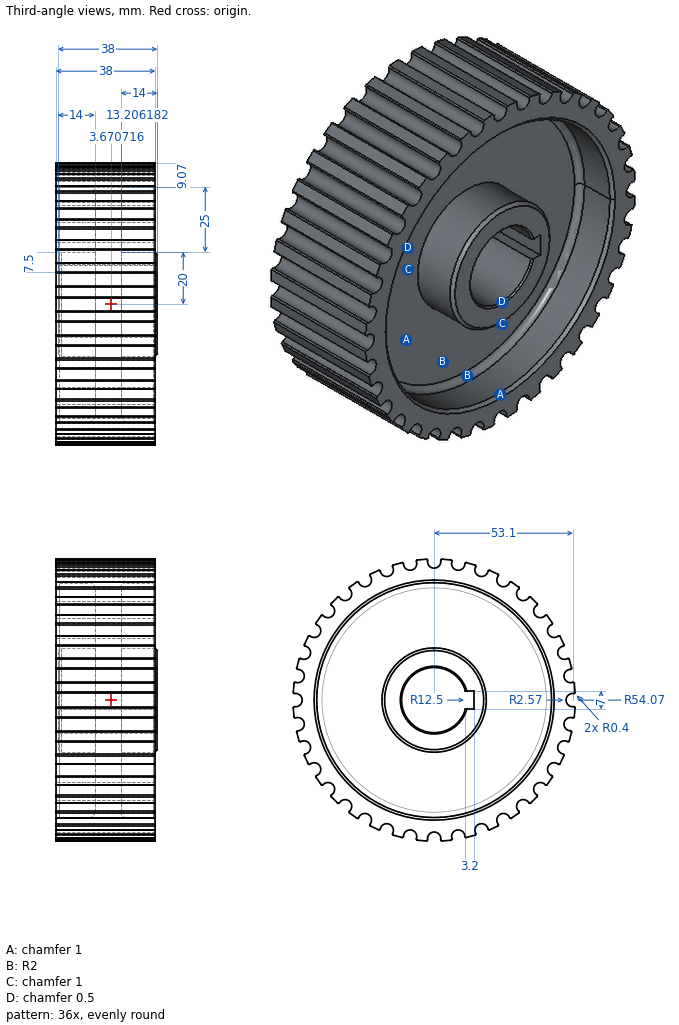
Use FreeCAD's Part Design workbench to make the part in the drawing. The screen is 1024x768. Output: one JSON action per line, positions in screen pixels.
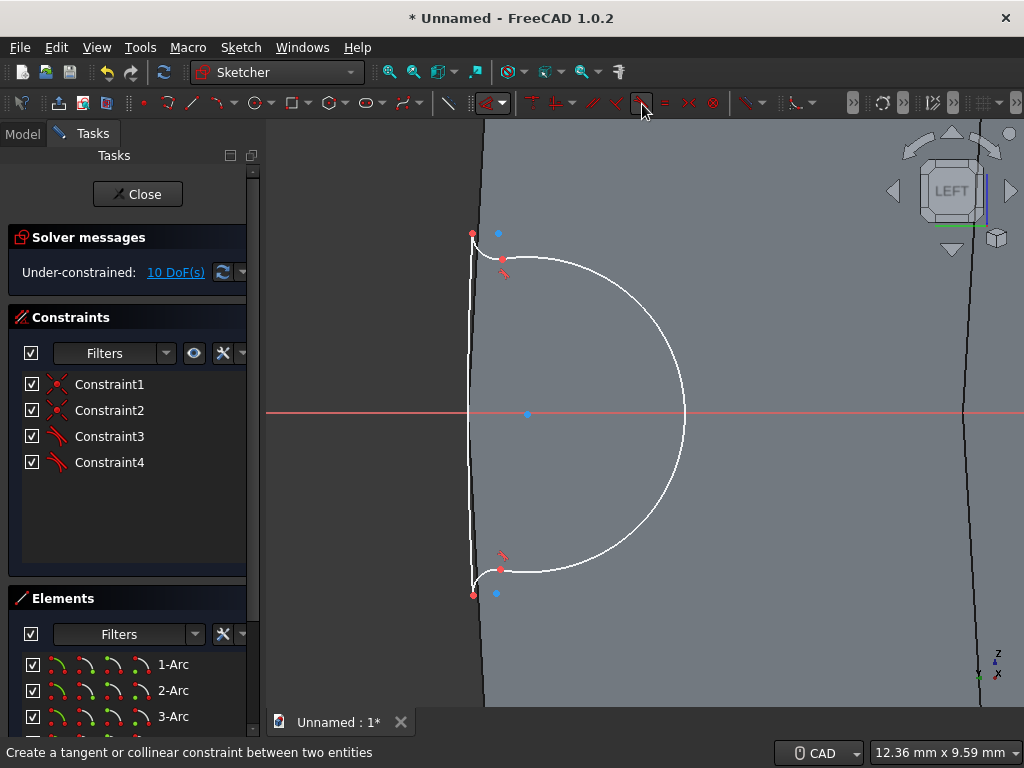
{"action": "left_click", "coordinate": [489, 258]}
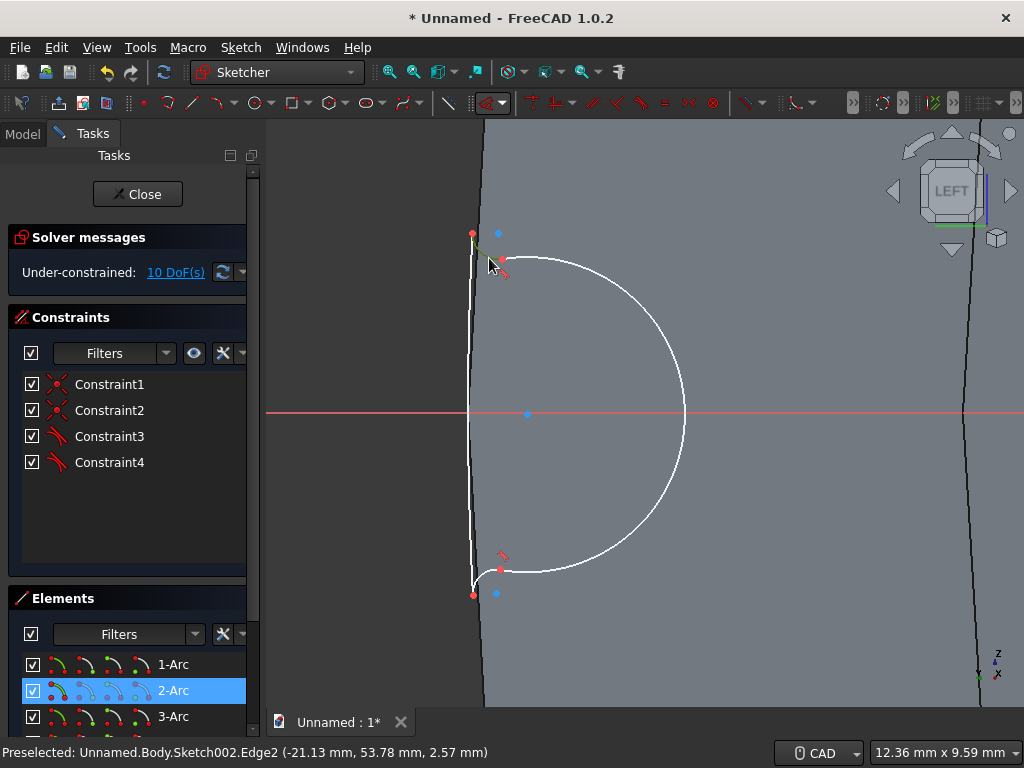
{"action": "left_click", "coordinate": [469, 342]}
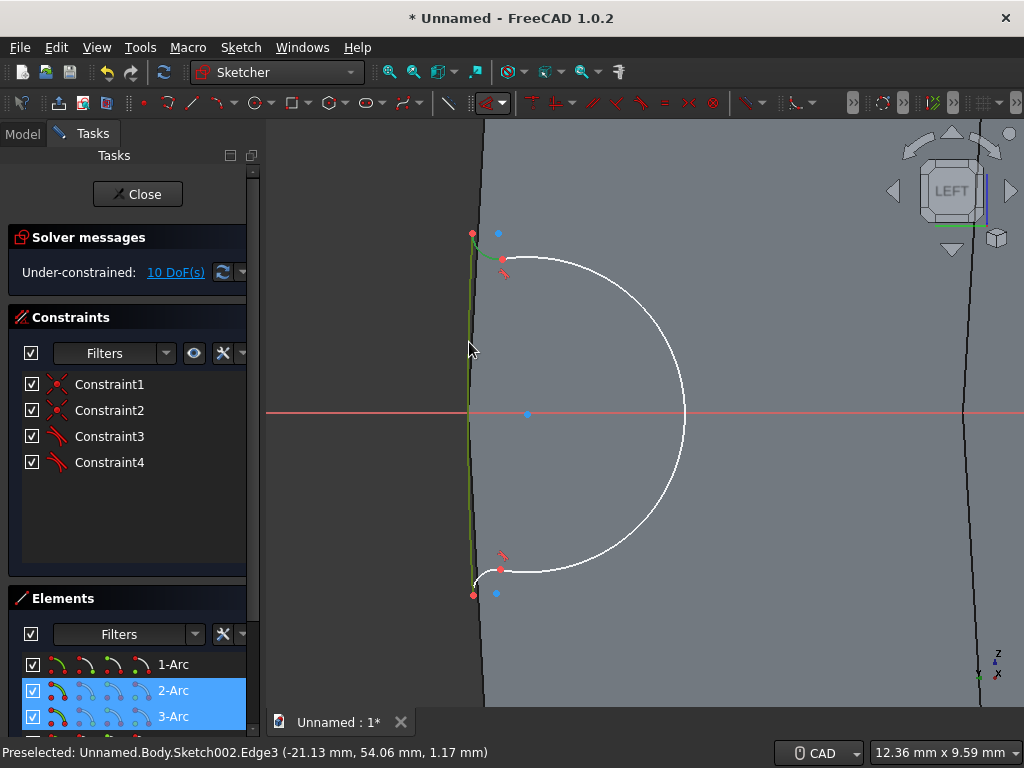
{"action": "key", "text": "t"}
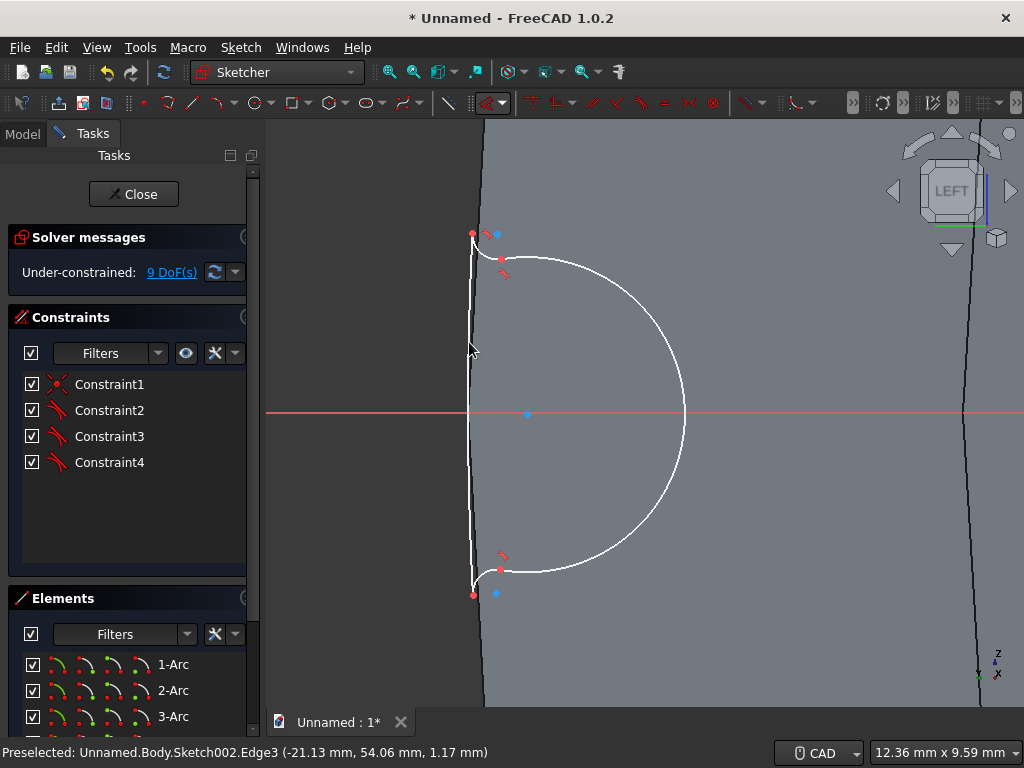
{"action": "left_click", "coordinate": [469, 342]}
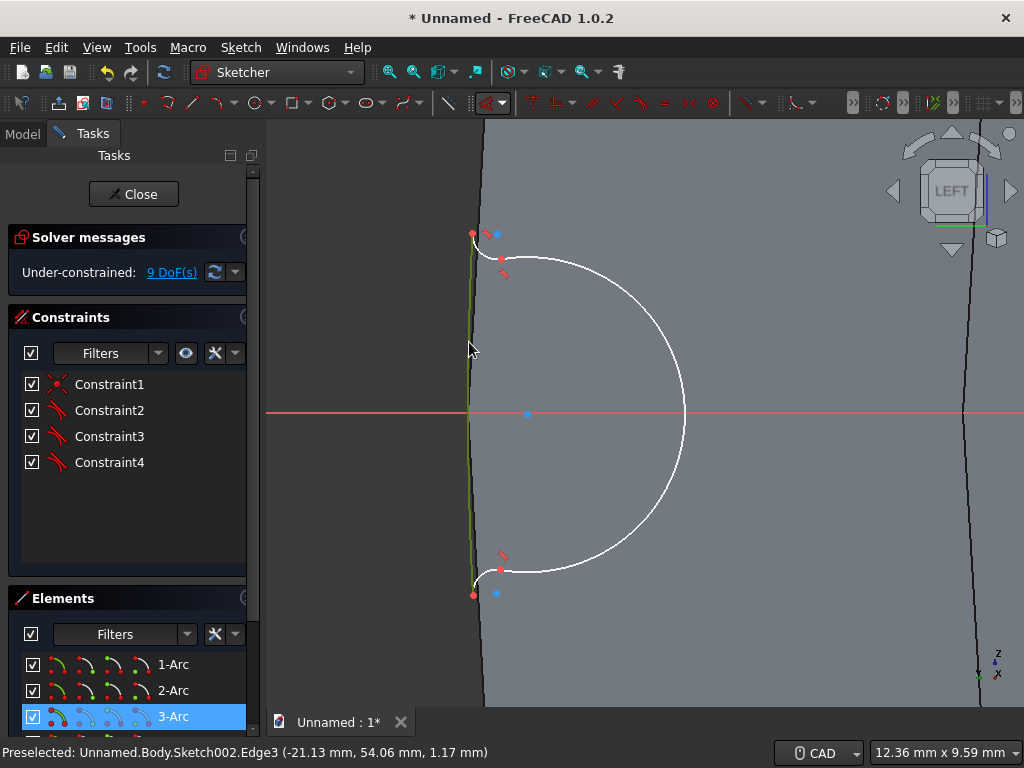
{"action": "left_click", "coordinate": [488, 571]}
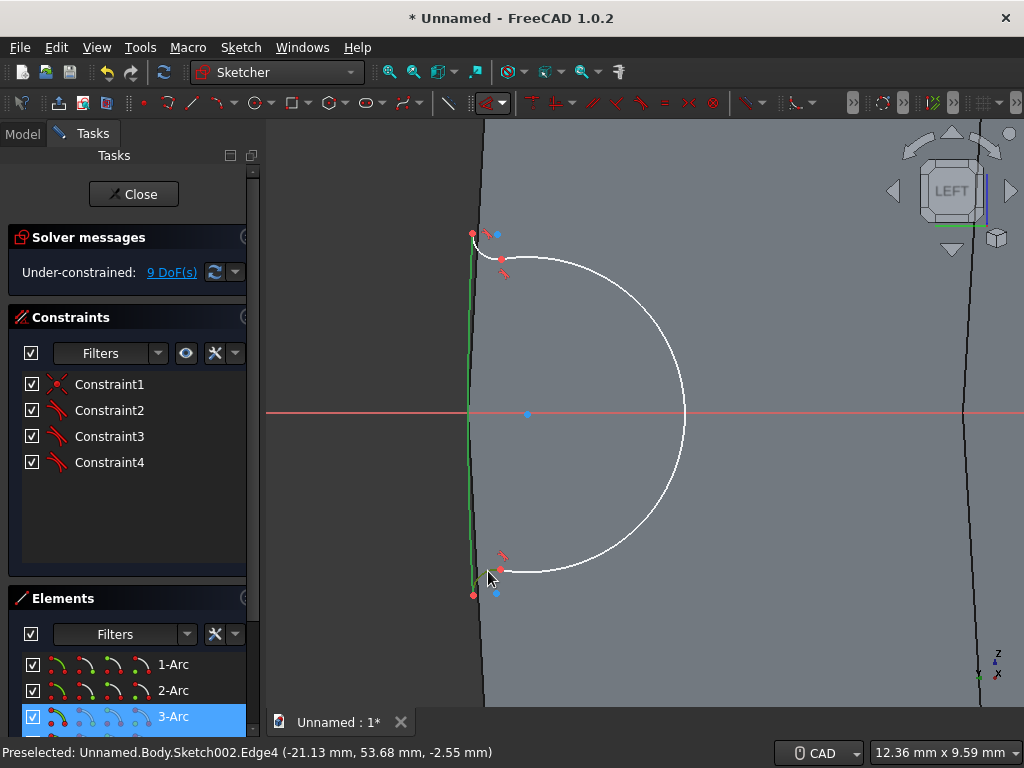
{"action": "key", "text": "t"}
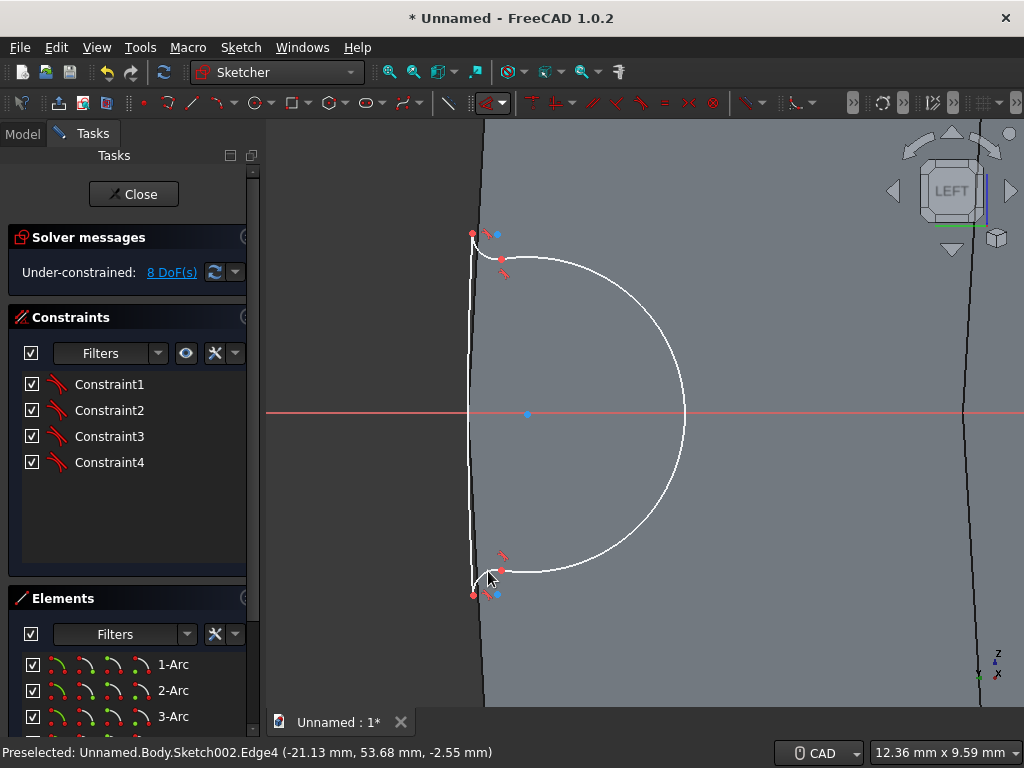
{"action": "scroll", "coordinate": [378, 413], "scroll_direction": "down", "scroll_amount": 11}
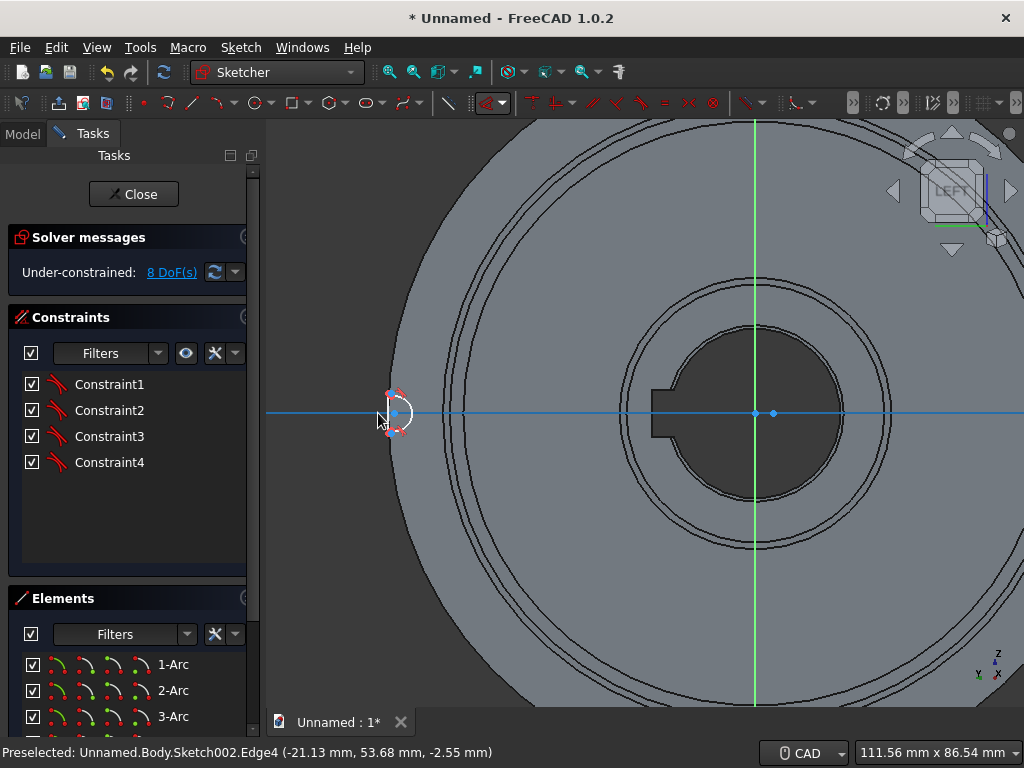
{"action": "scroll", "coordinate": [764, 413], "scroll_direction": "up", "scroll_amount": 14}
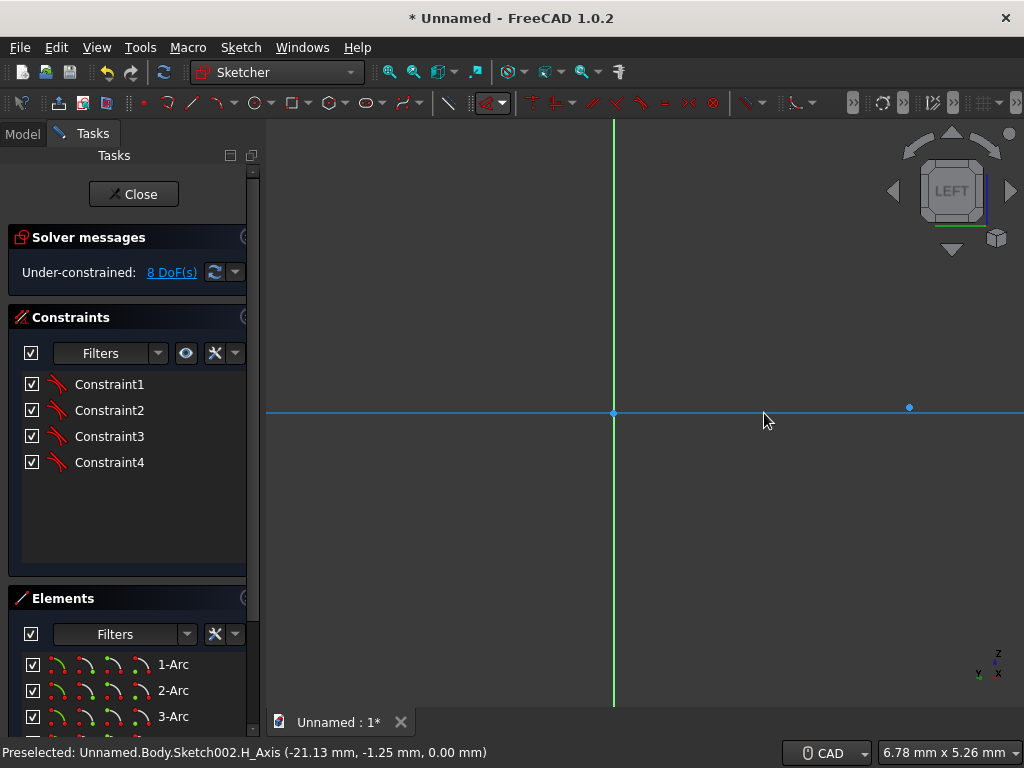
{"action": "left_click_drag", "start_coordinate": [604, 397], "coordinate": [919, 423]}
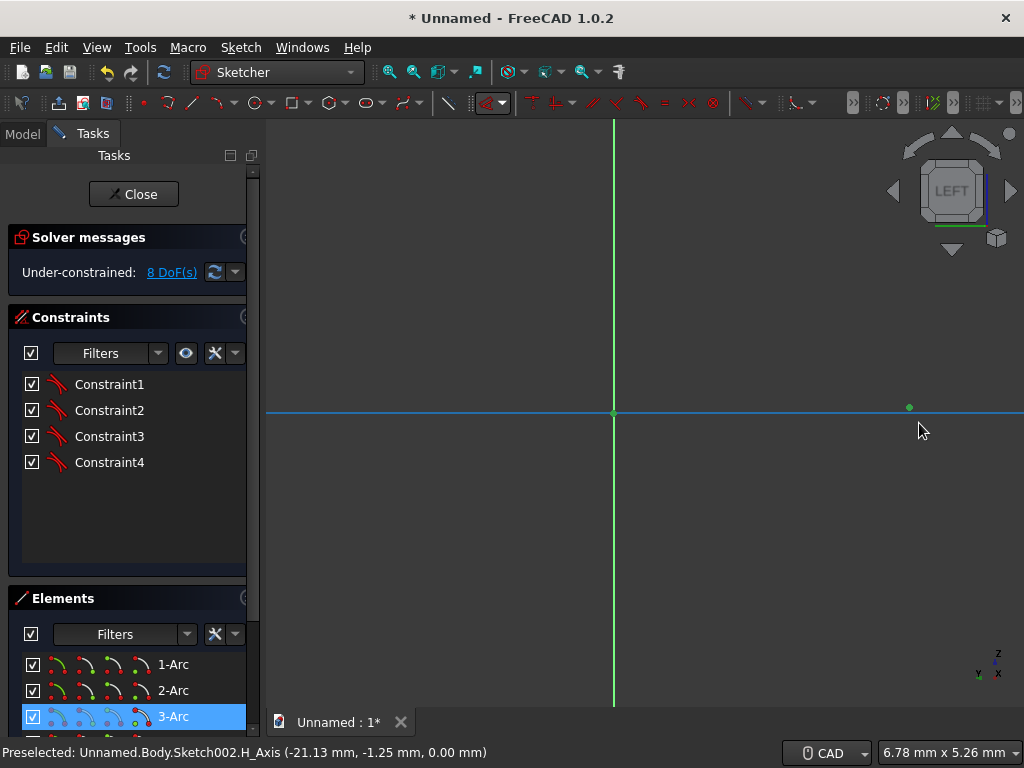
{"action": "left_click", "coordinate": [532, 104]}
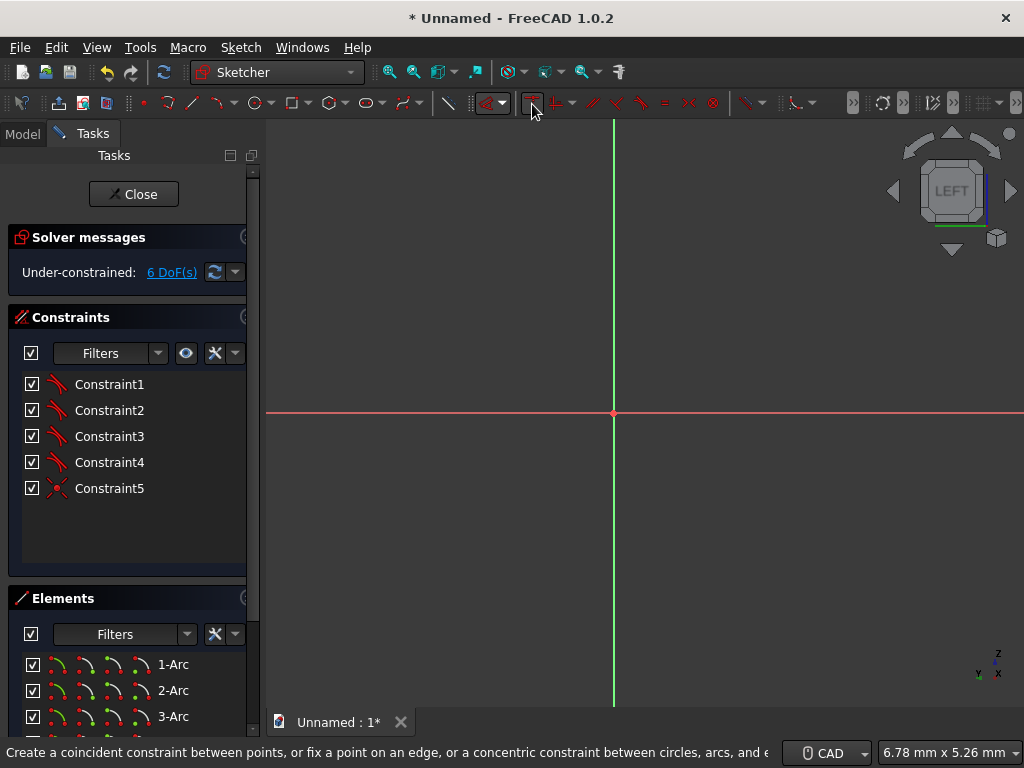
{"action": "scroll", "coordinate": [576, 413], "scroll_direction": "down", "scroll_amount": 5}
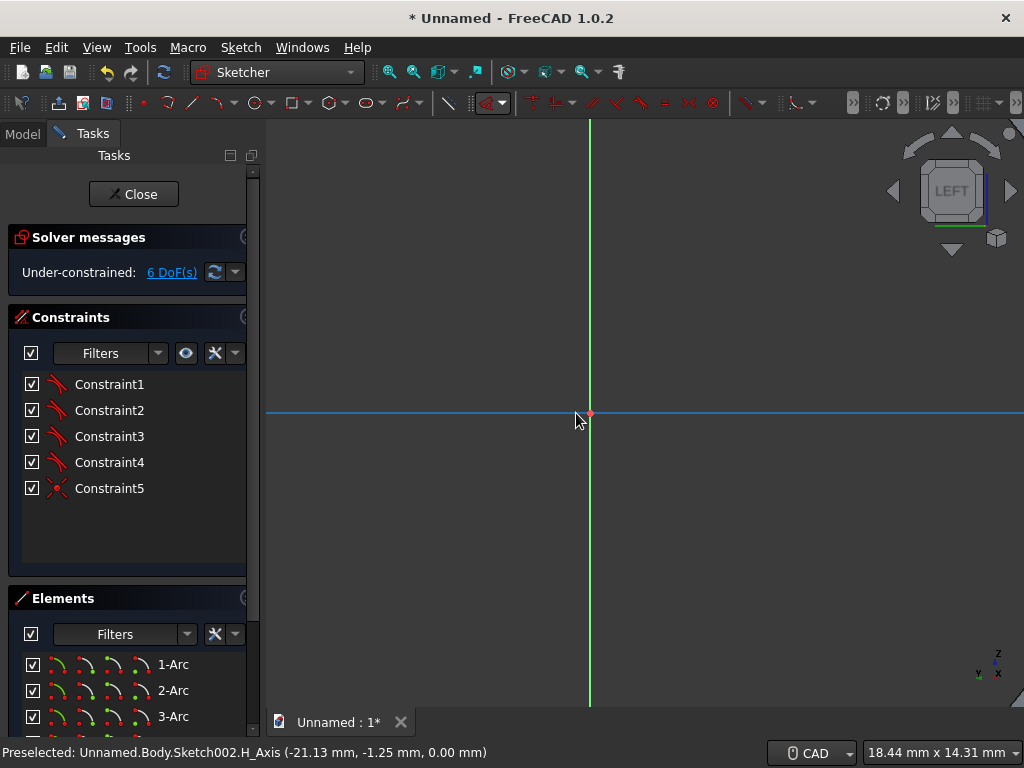
{"action": "scroll", "coordinate": [576, 413], "scroll_direction": "down", "scroll_amount": 5}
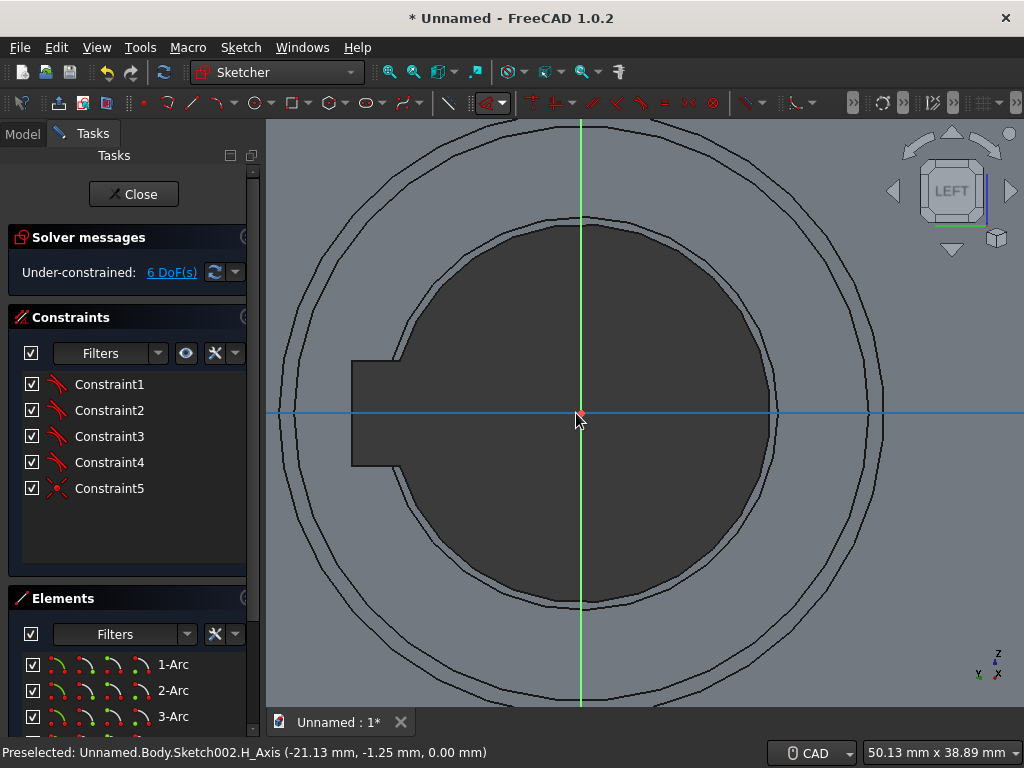
{"action": "scroll", "coordinate": [576, 413], "scroll_direction": "down", "scroll_amount": 5}